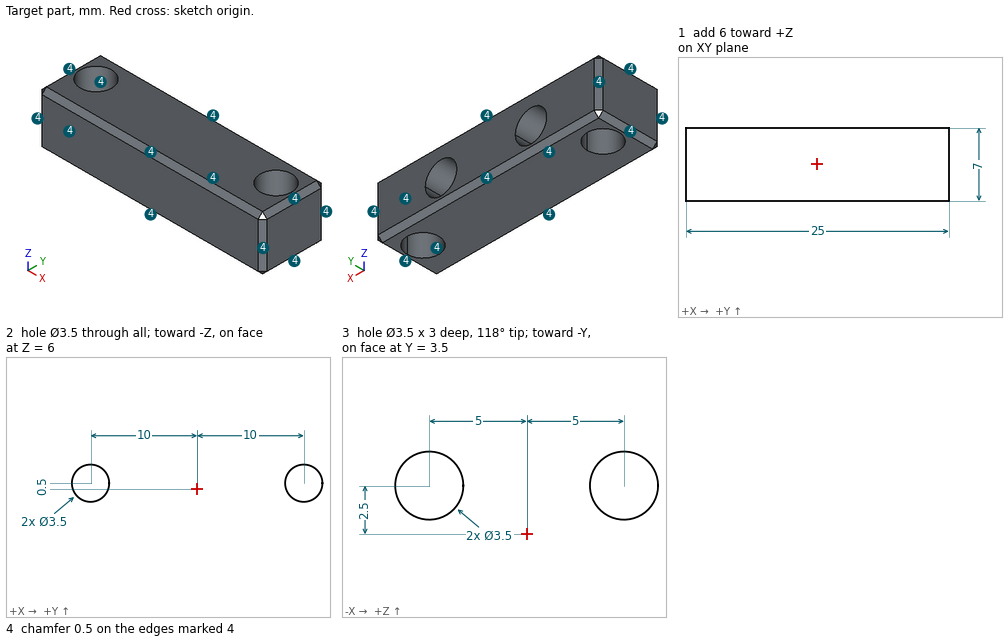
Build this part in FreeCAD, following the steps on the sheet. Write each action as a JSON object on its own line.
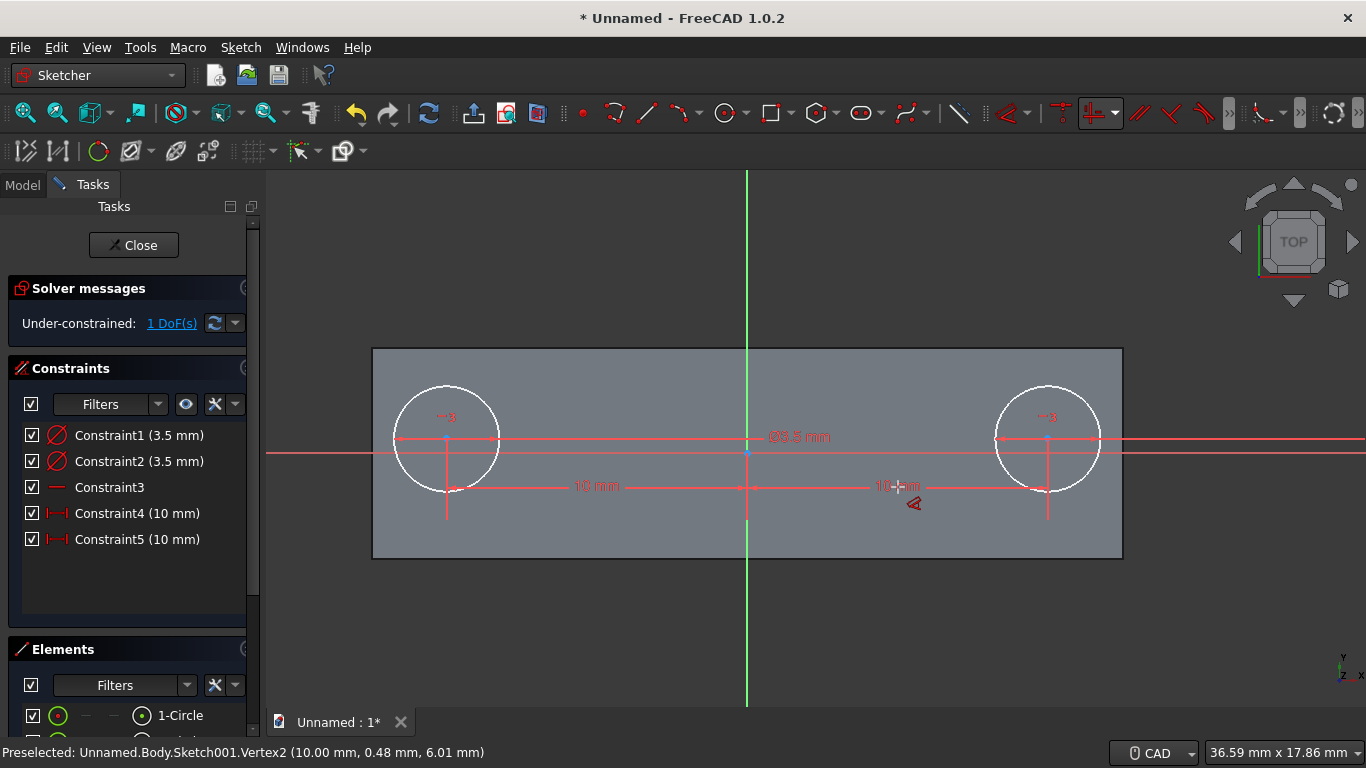
{"action": "scroll", "coordinate": [447, 439], "scroll_direction": "up", "scroll_amount": 5}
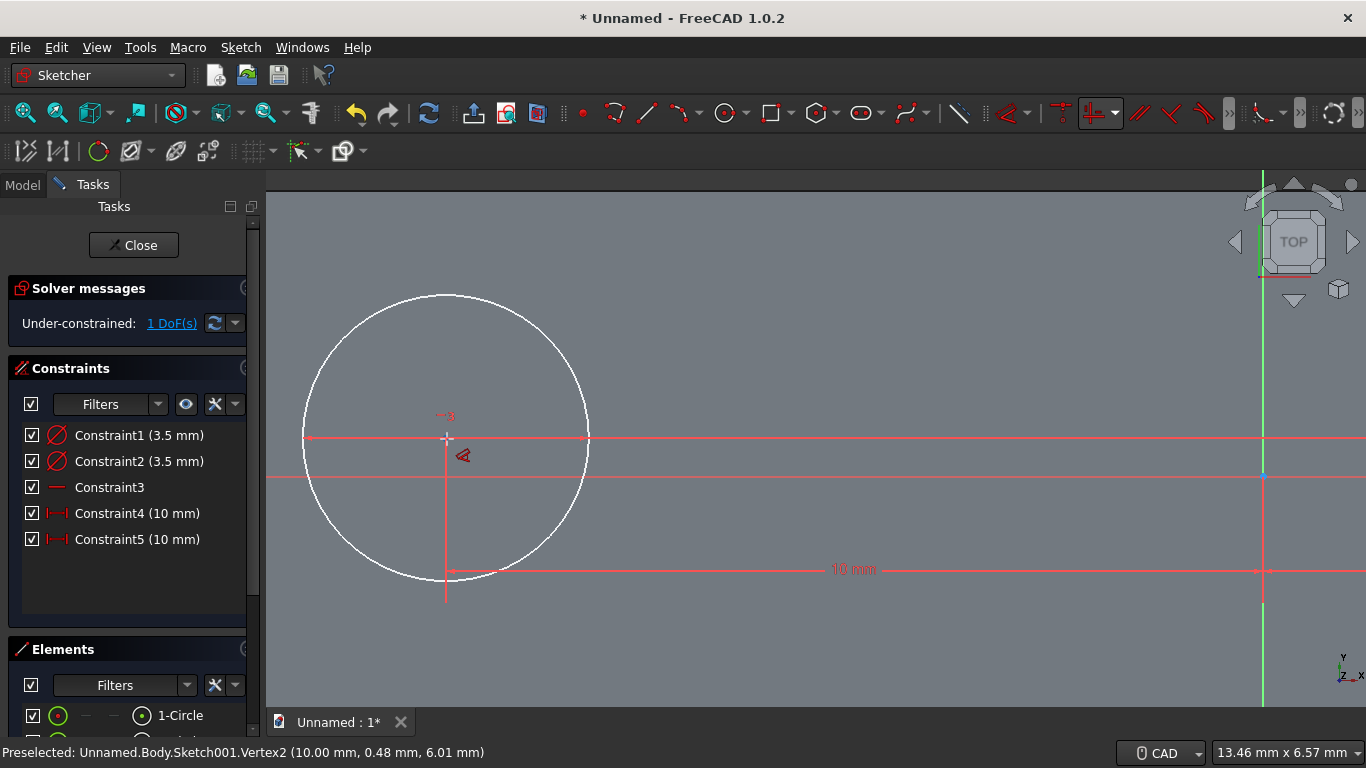
{"action": "left_click", "coordinate": [446, 438]}
{"action": "left_click", "coordinate": [412, 458]}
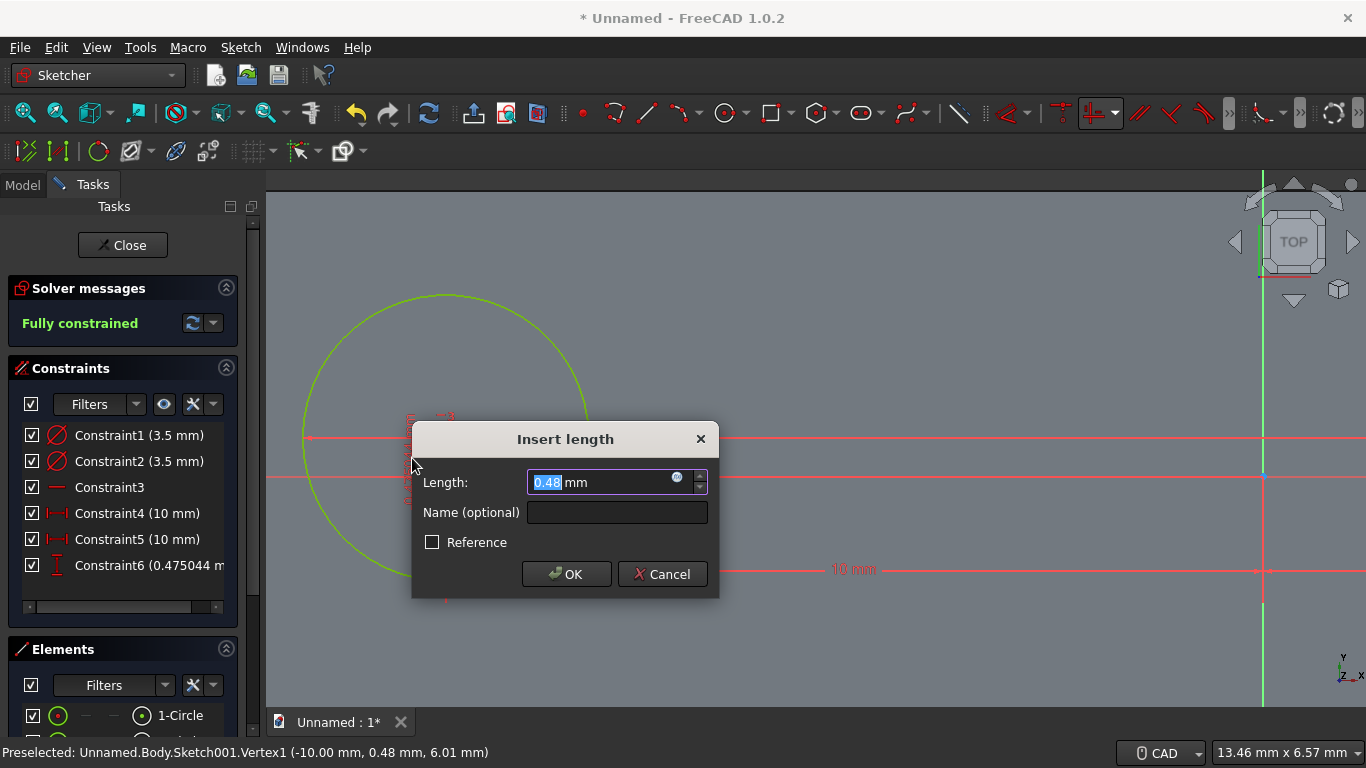
{"action": "type", "text": "0.5"}
{"action": "key", "text": "Return"}
{"action": "key", "text": "Escape"}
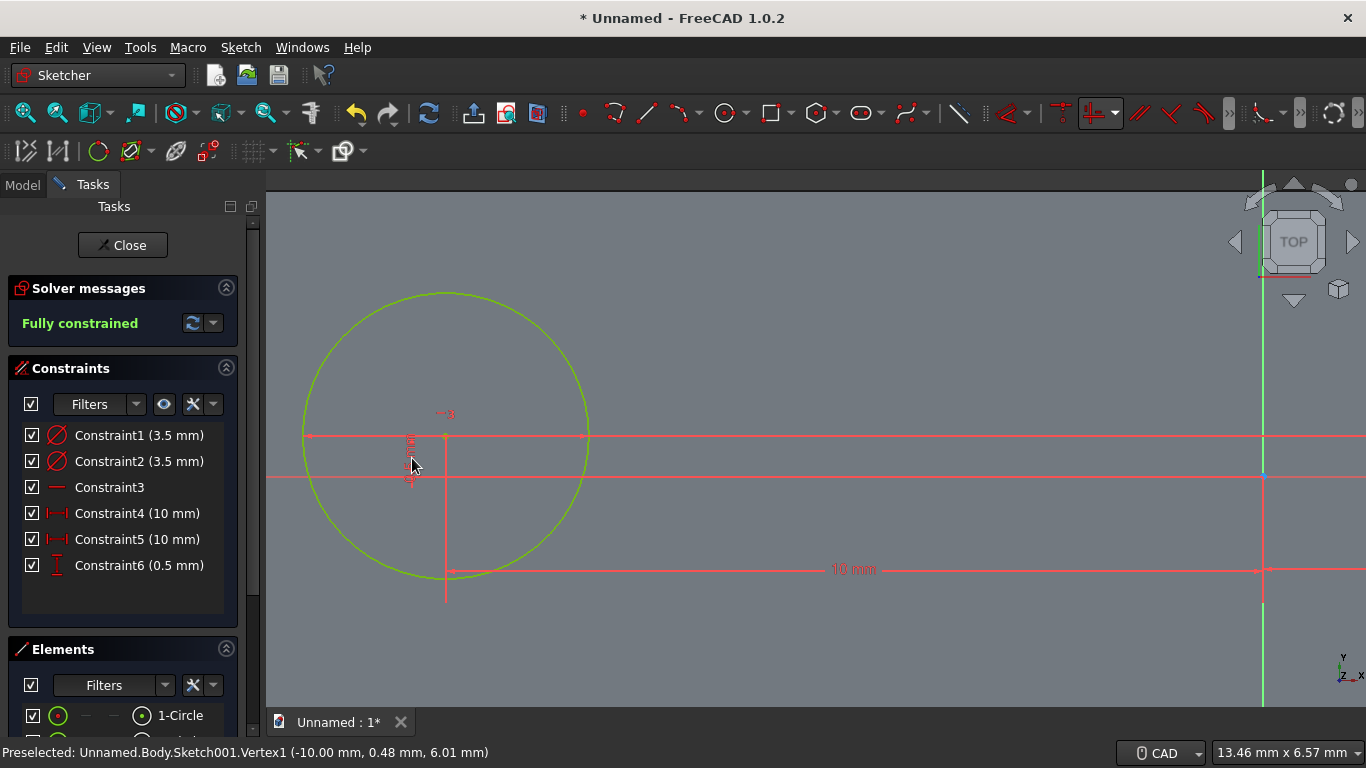
{"action": "left_click", "coordinate": [123, 245]}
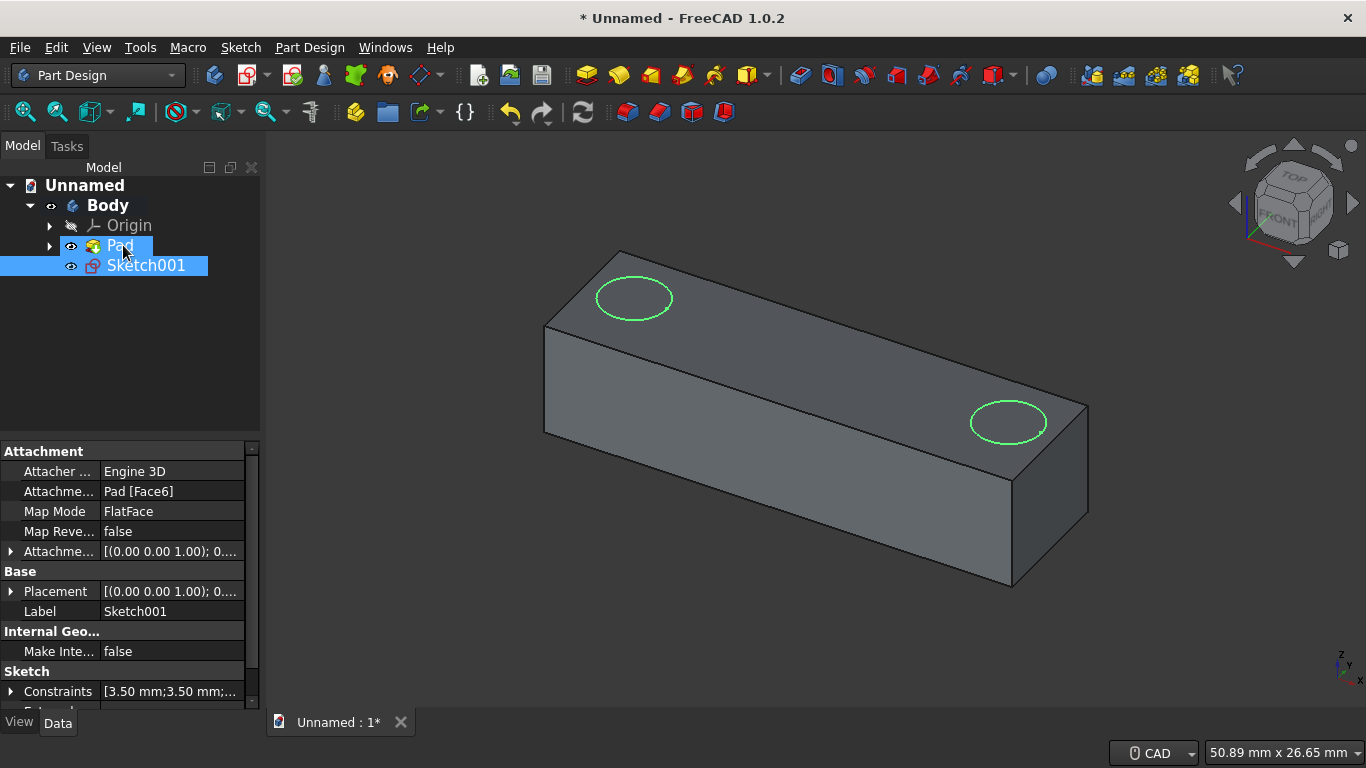
{"action": "left_click", "coordinate": [834, 76]}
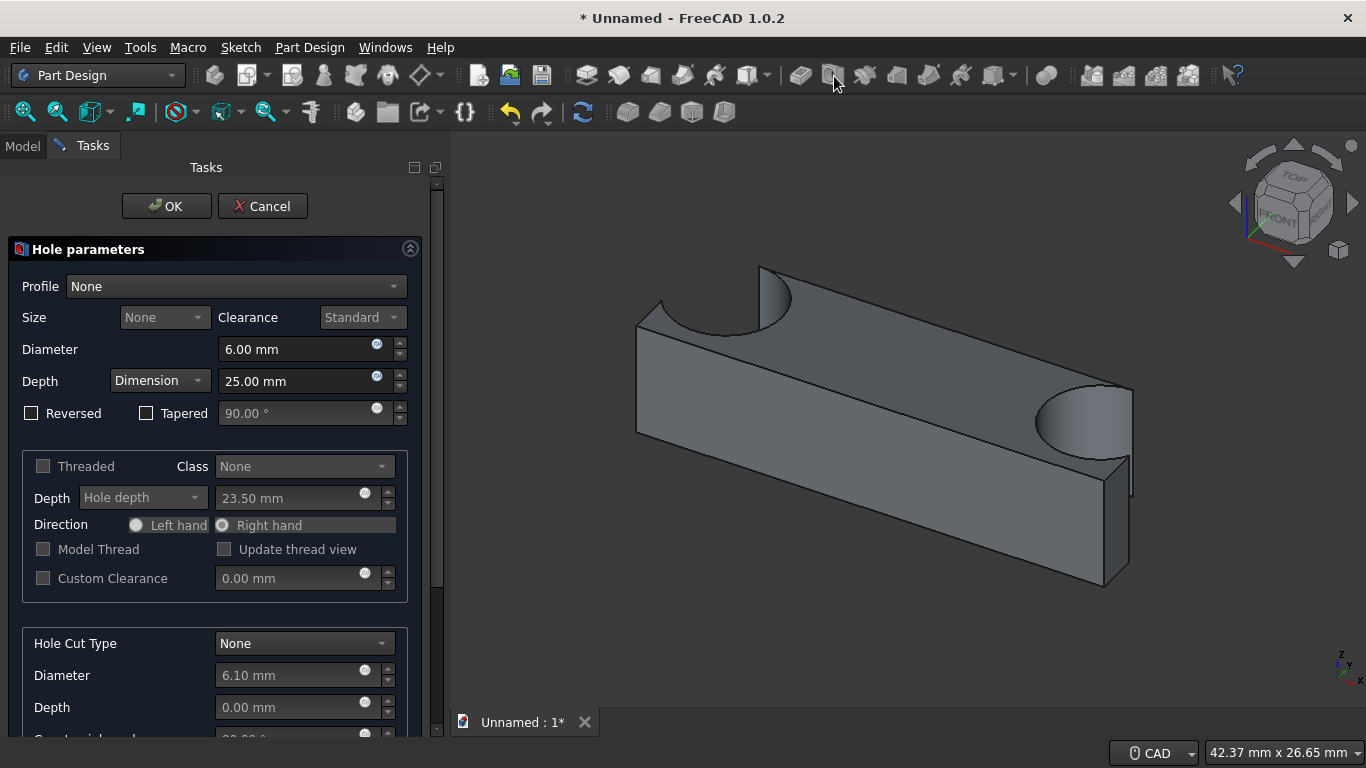
{"action": "triple_click", "coordinate": [305, 349]}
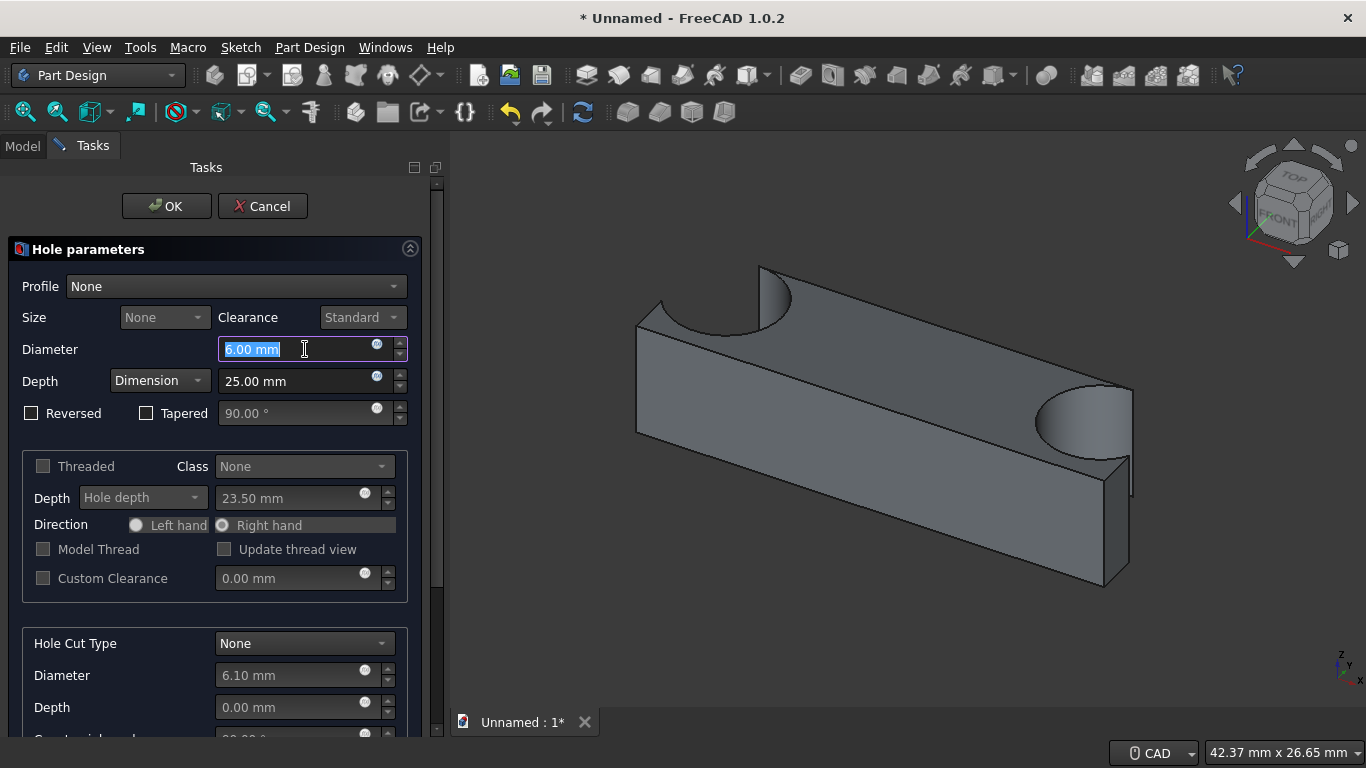
{"action": "type", "text": "3.5"}
{"action": "key", "text": "Tab"}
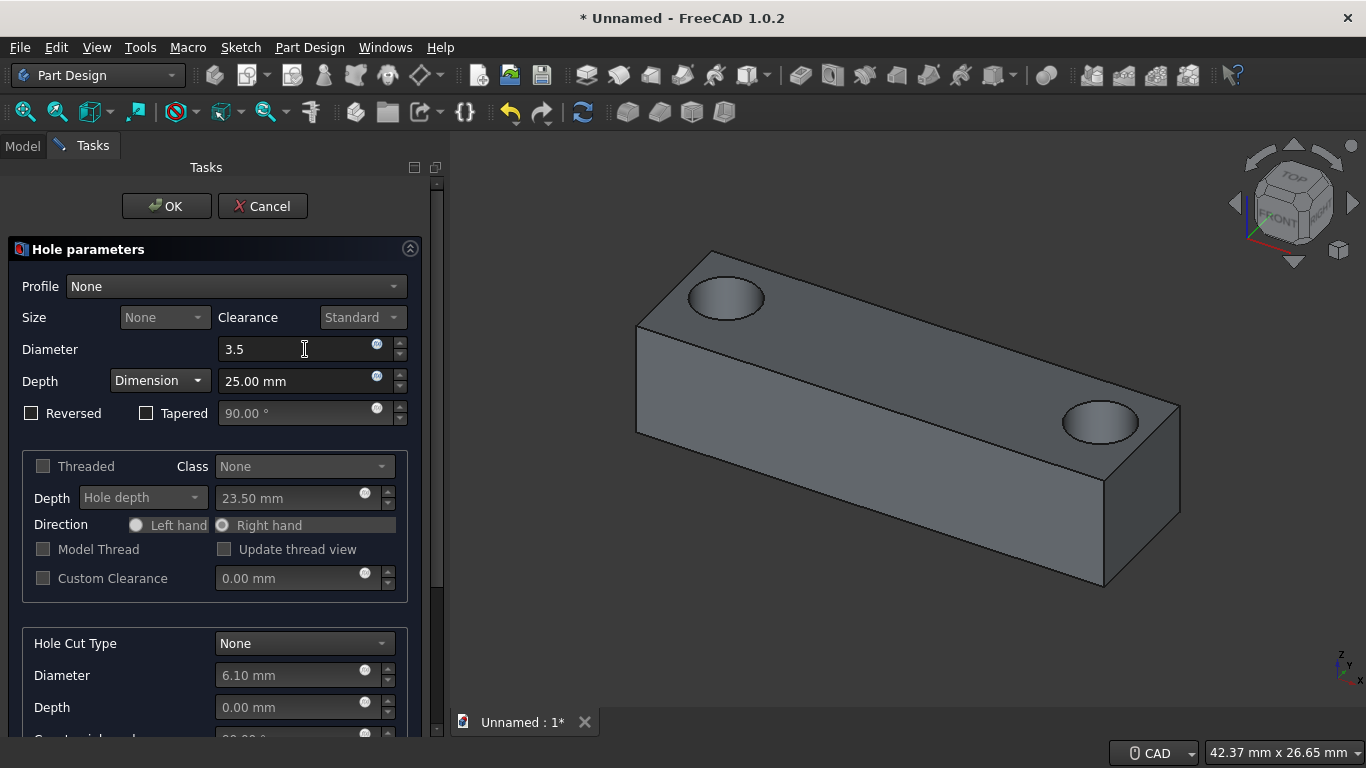
{"action": "left_click", "coordinate": [161, 380]}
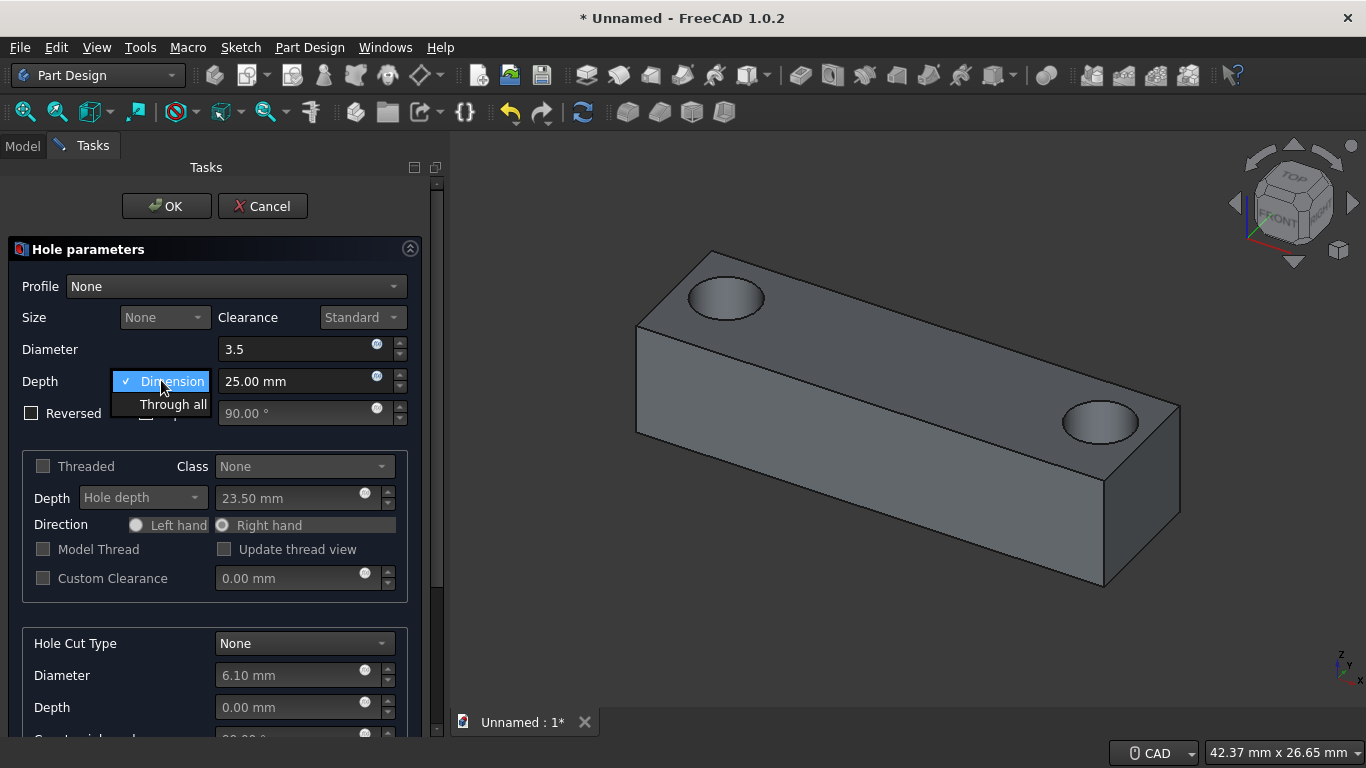
{"action": "left_click", "coordinate": [160, 404]}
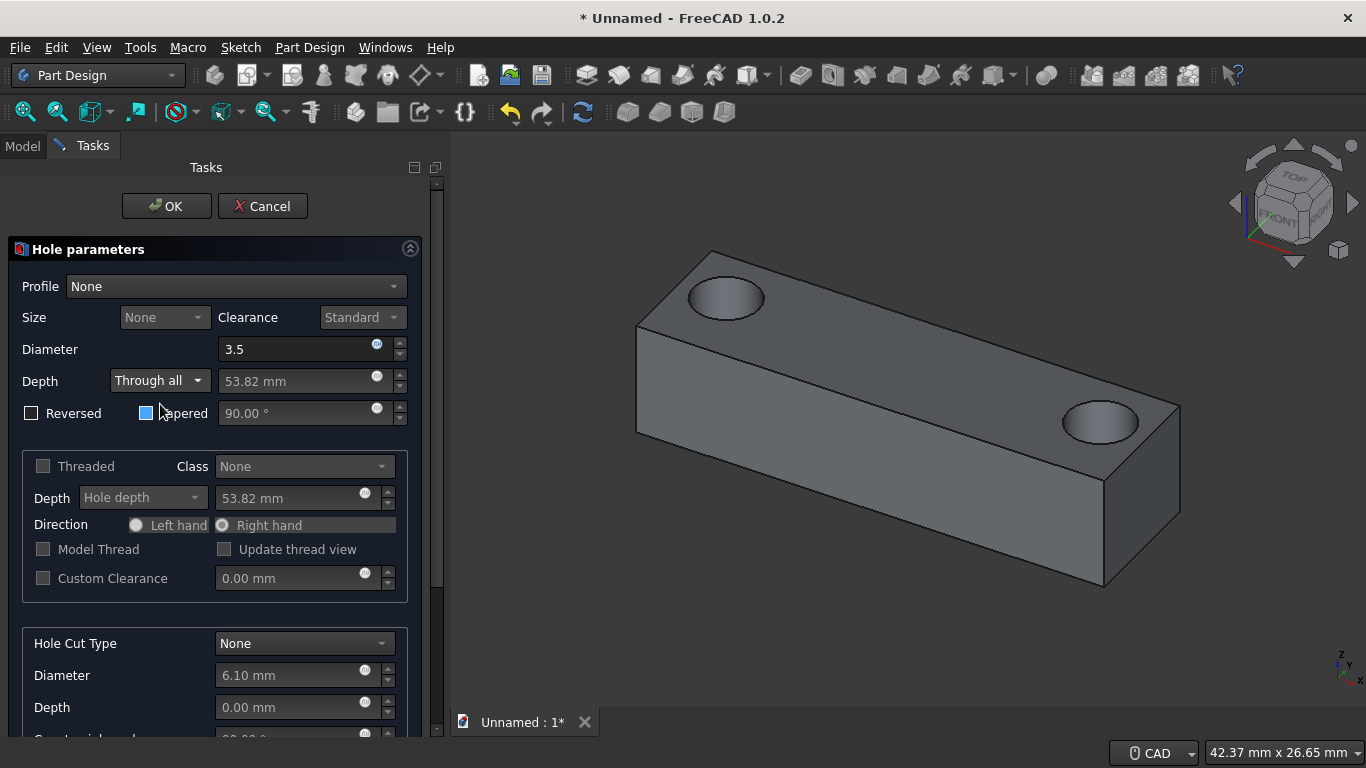
{"action": "left_click", "coordinate": [167, 206]}